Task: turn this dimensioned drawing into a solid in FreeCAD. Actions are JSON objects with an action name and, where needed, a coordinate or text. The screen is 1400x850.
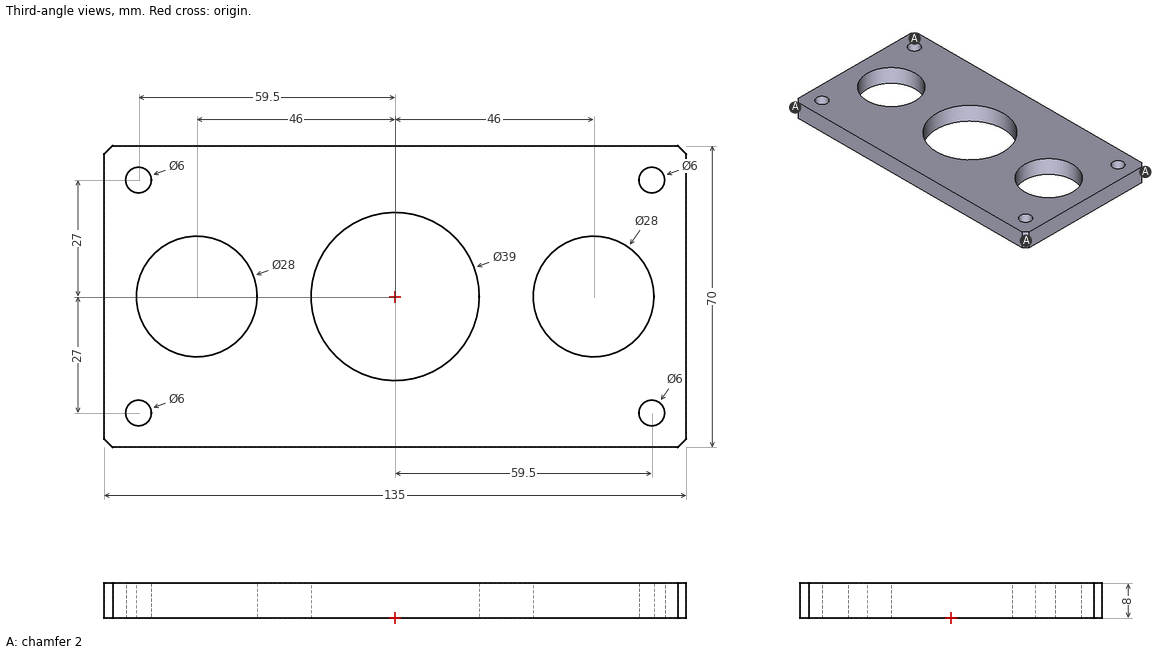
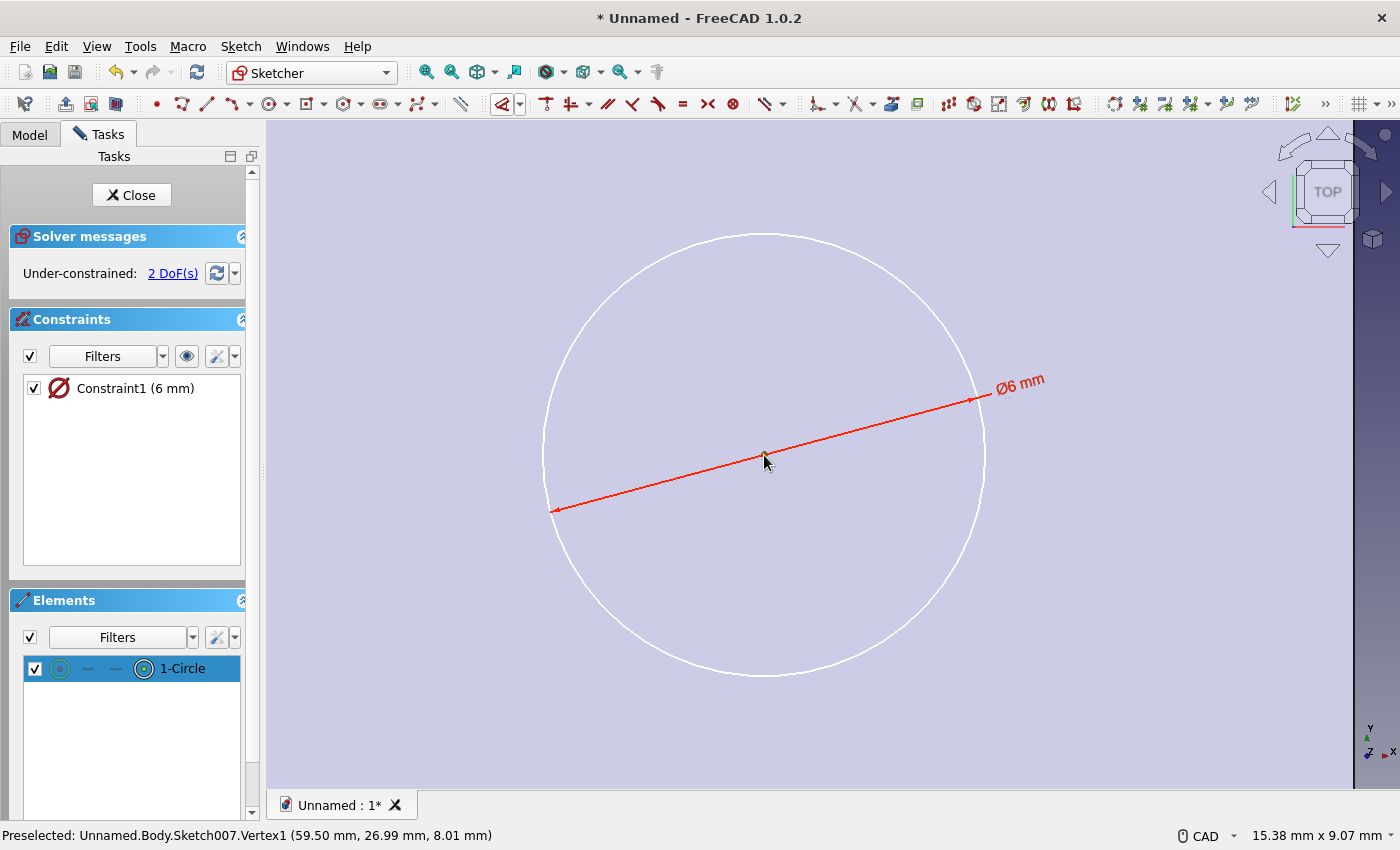
{"action": "key", "text": "i"}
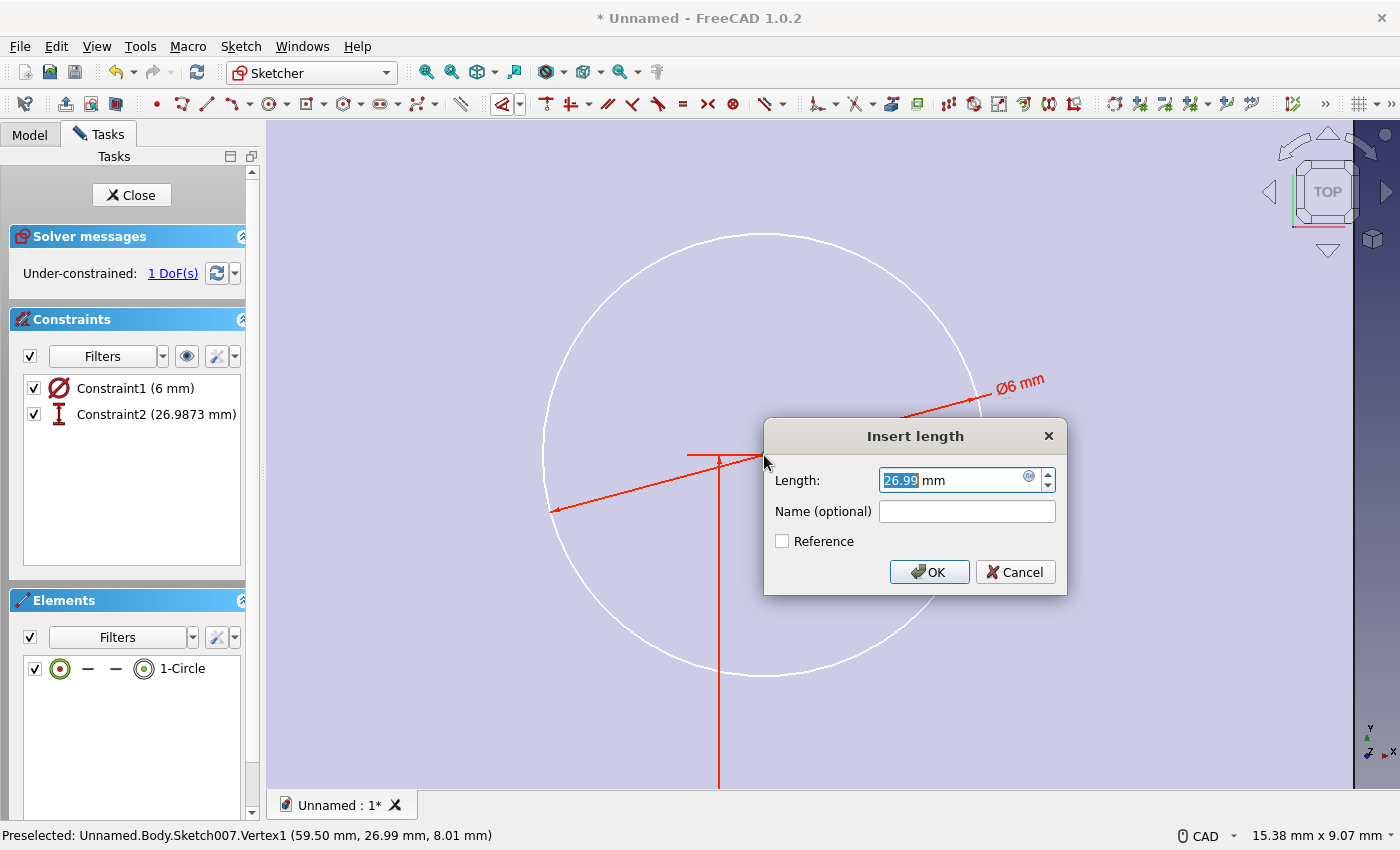
{"action": "type", "text": "27"}
{"action": "key", "text": "Return"}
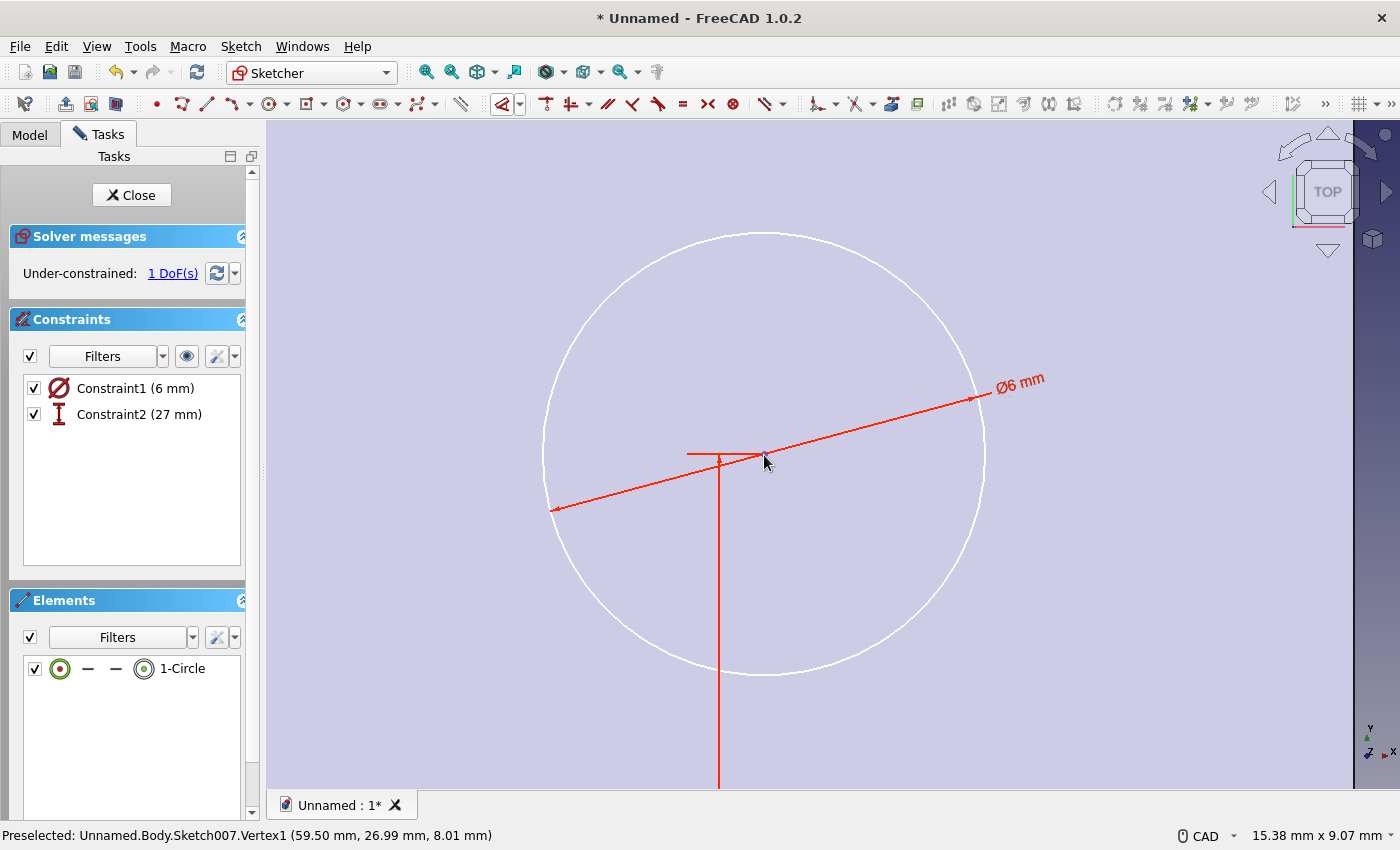
{"action": "left_click", "coordinate": [764, 454]}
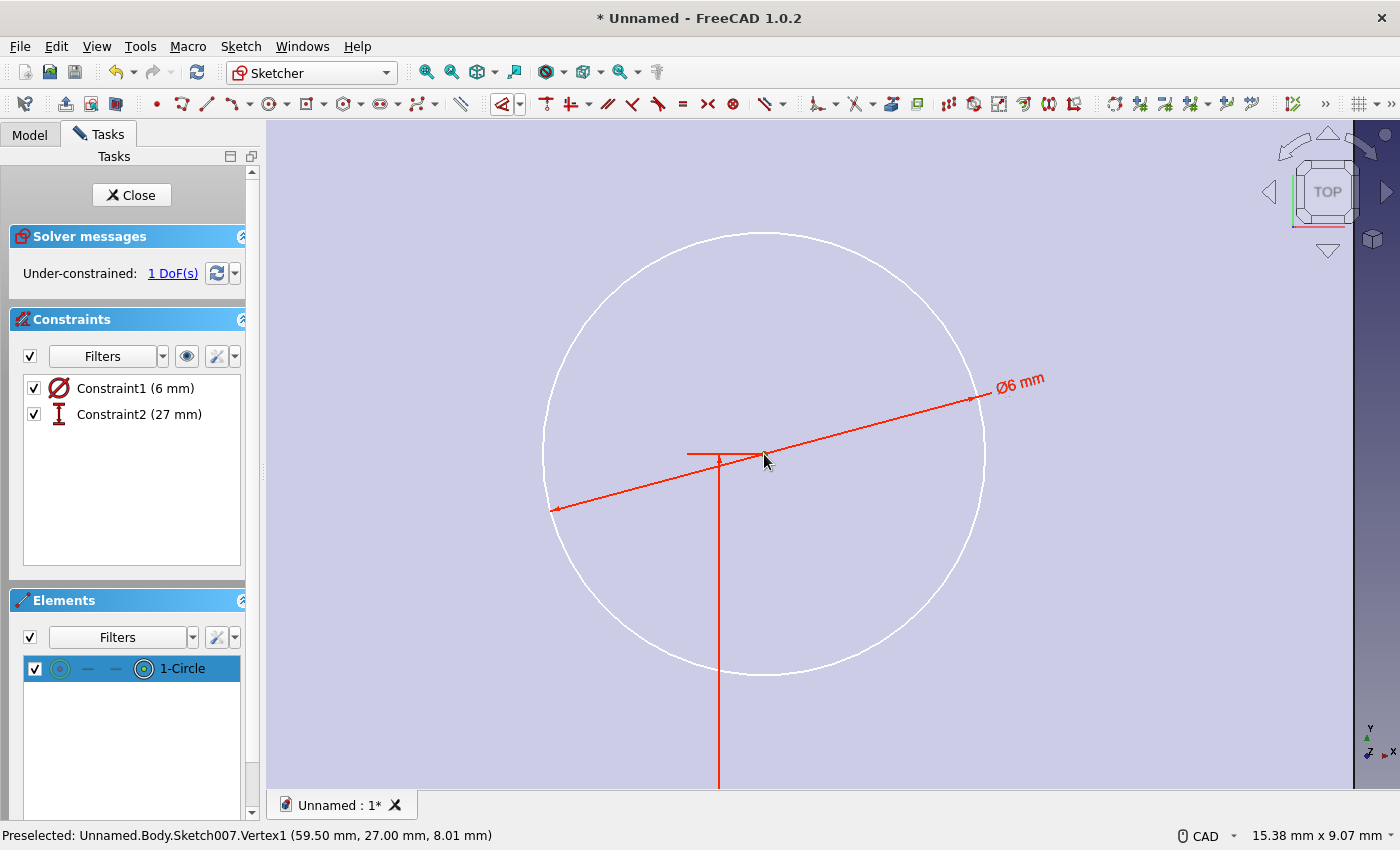
{"action": "key", "text": "l"}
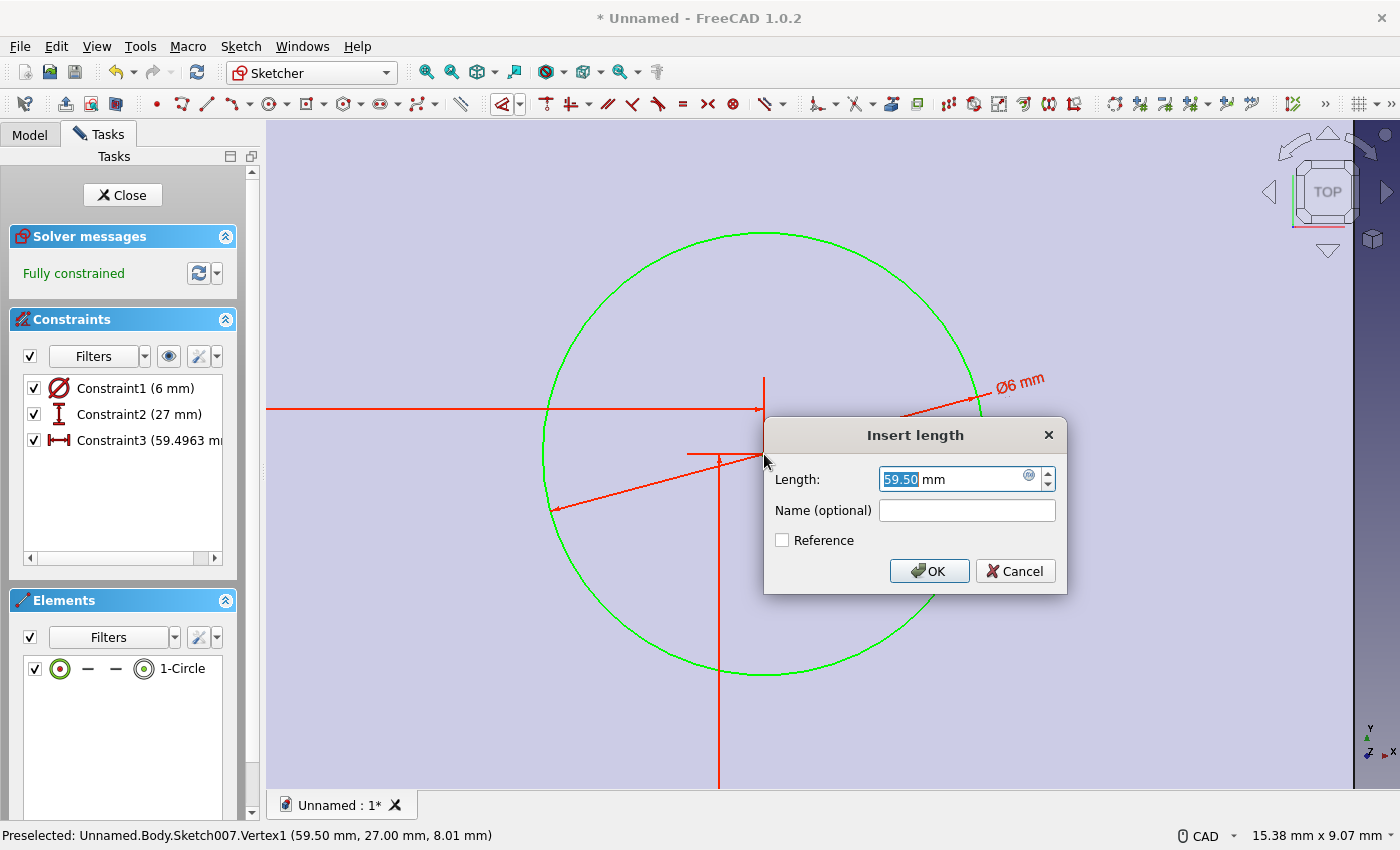
{"action": "type", "text": "59.5"}
{"action": "key", "text": "Return"}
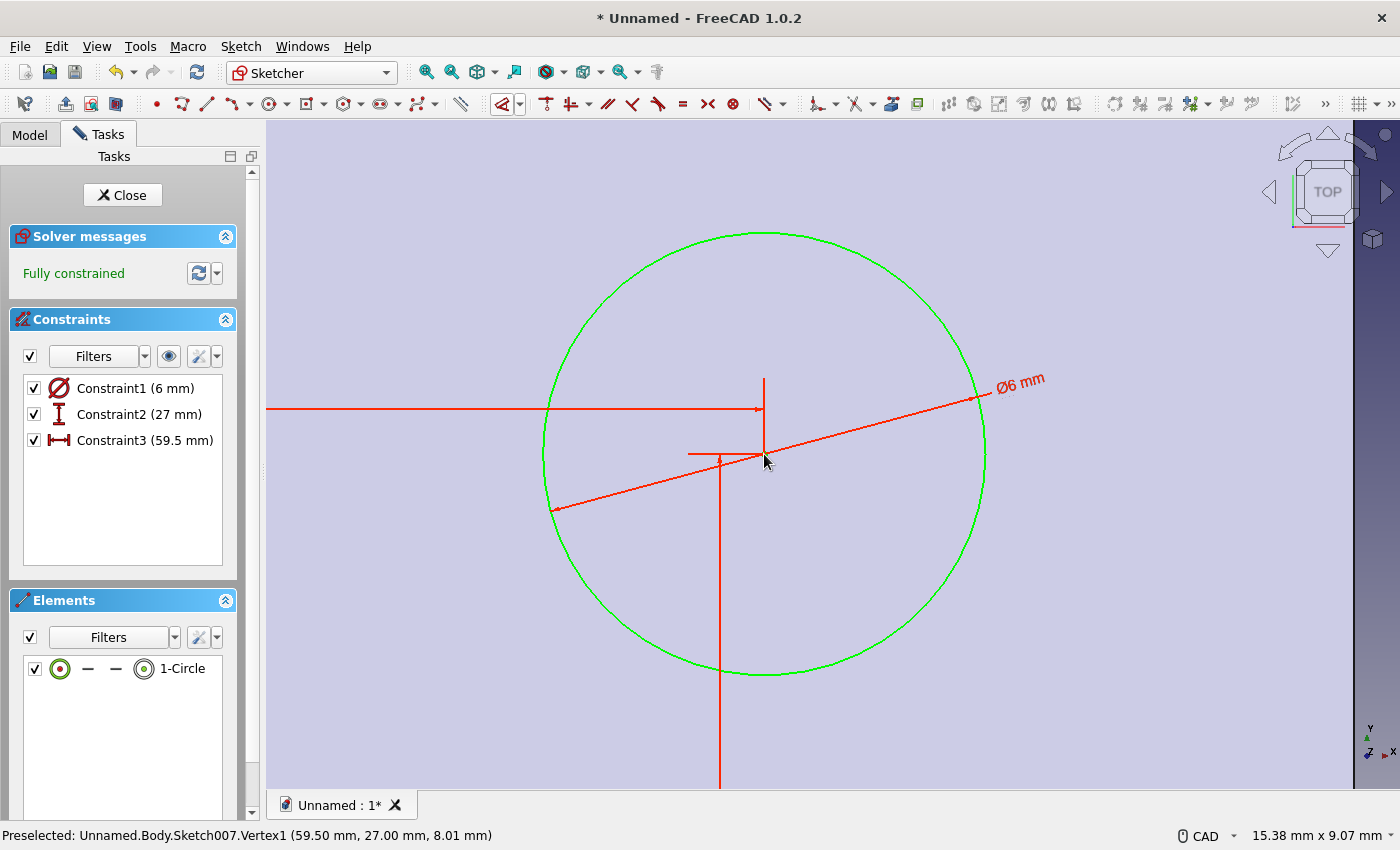
{"action": "left_click", "coordinate": [123, 195]}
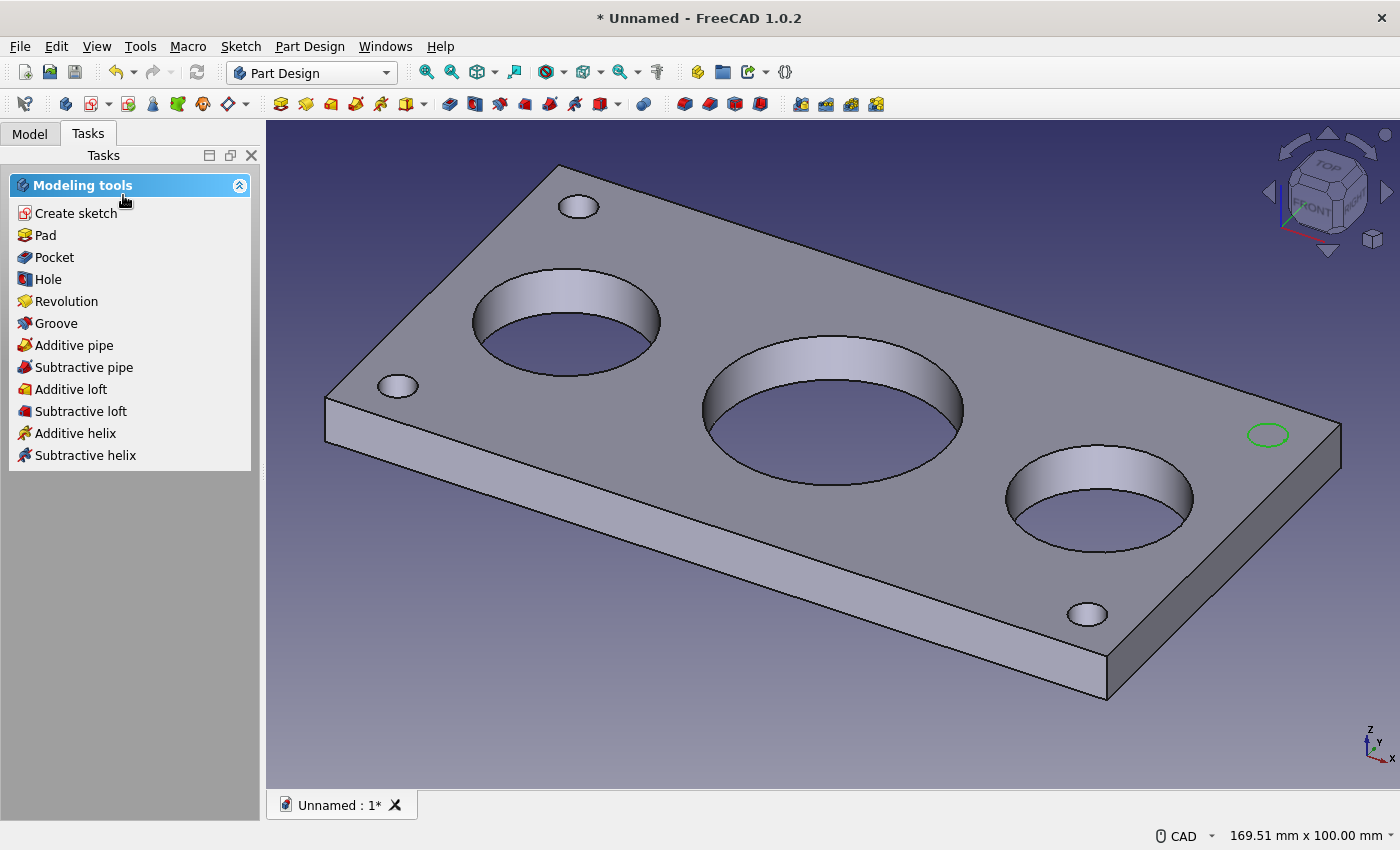
{"action": "left_click", "coordinate": [450, 104]}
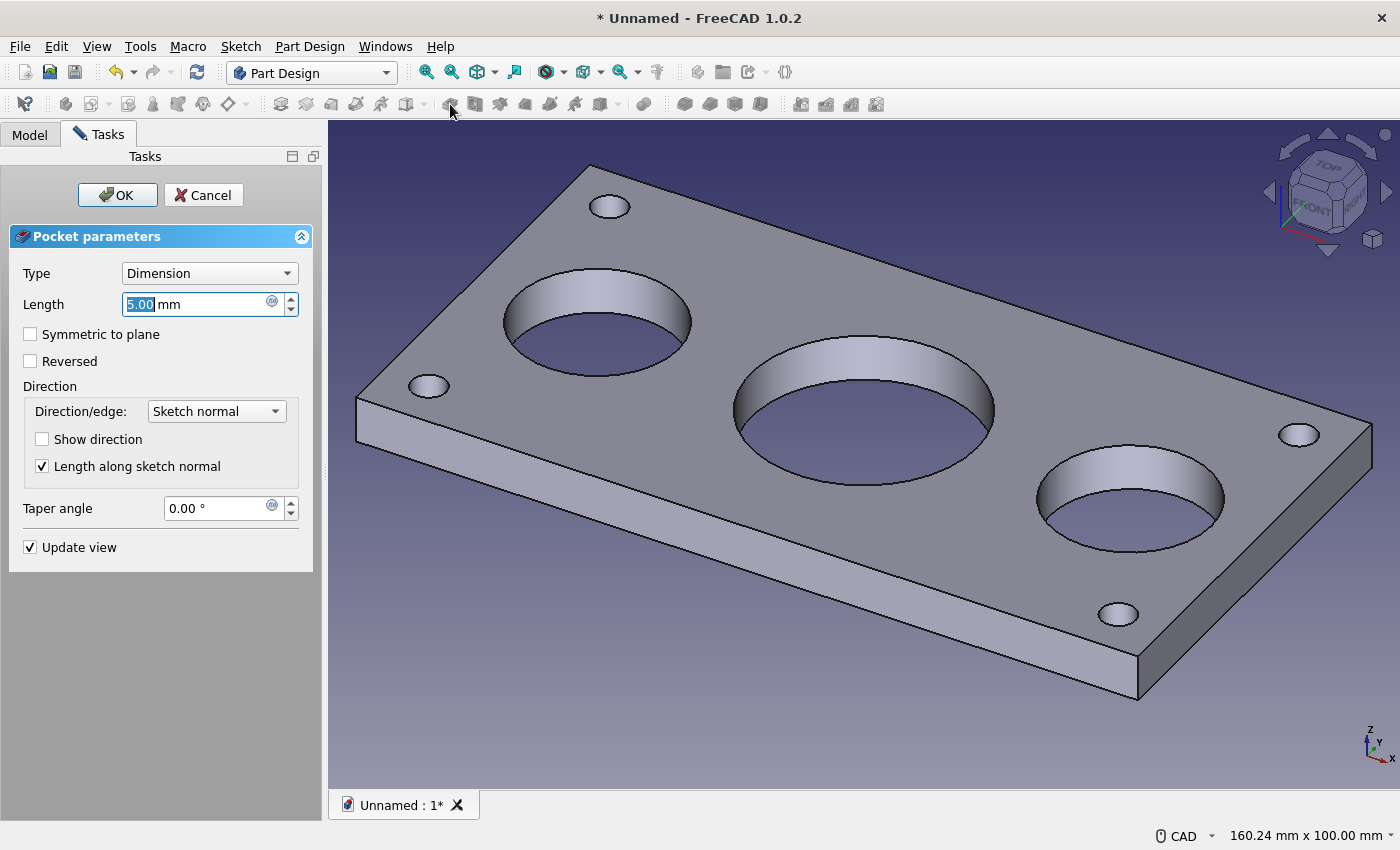
{"action": "left_click", "coordinate": [210, 274]}